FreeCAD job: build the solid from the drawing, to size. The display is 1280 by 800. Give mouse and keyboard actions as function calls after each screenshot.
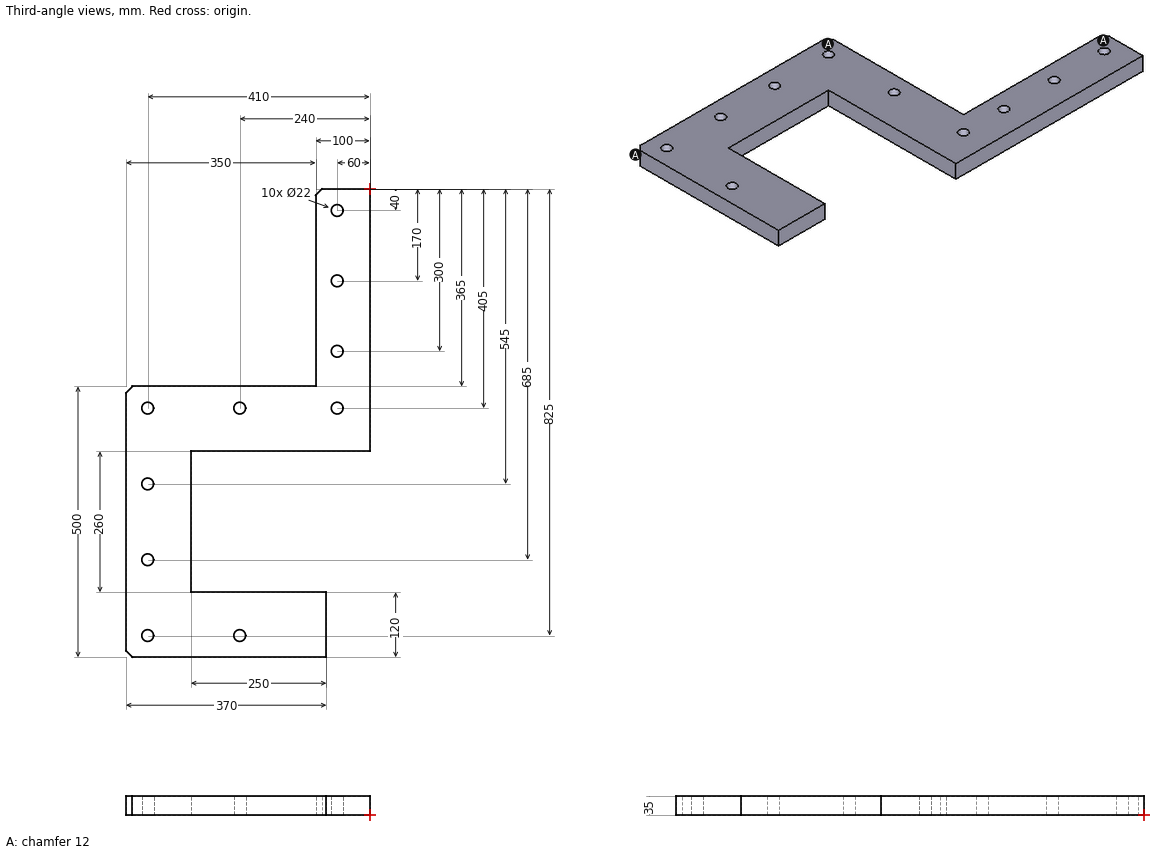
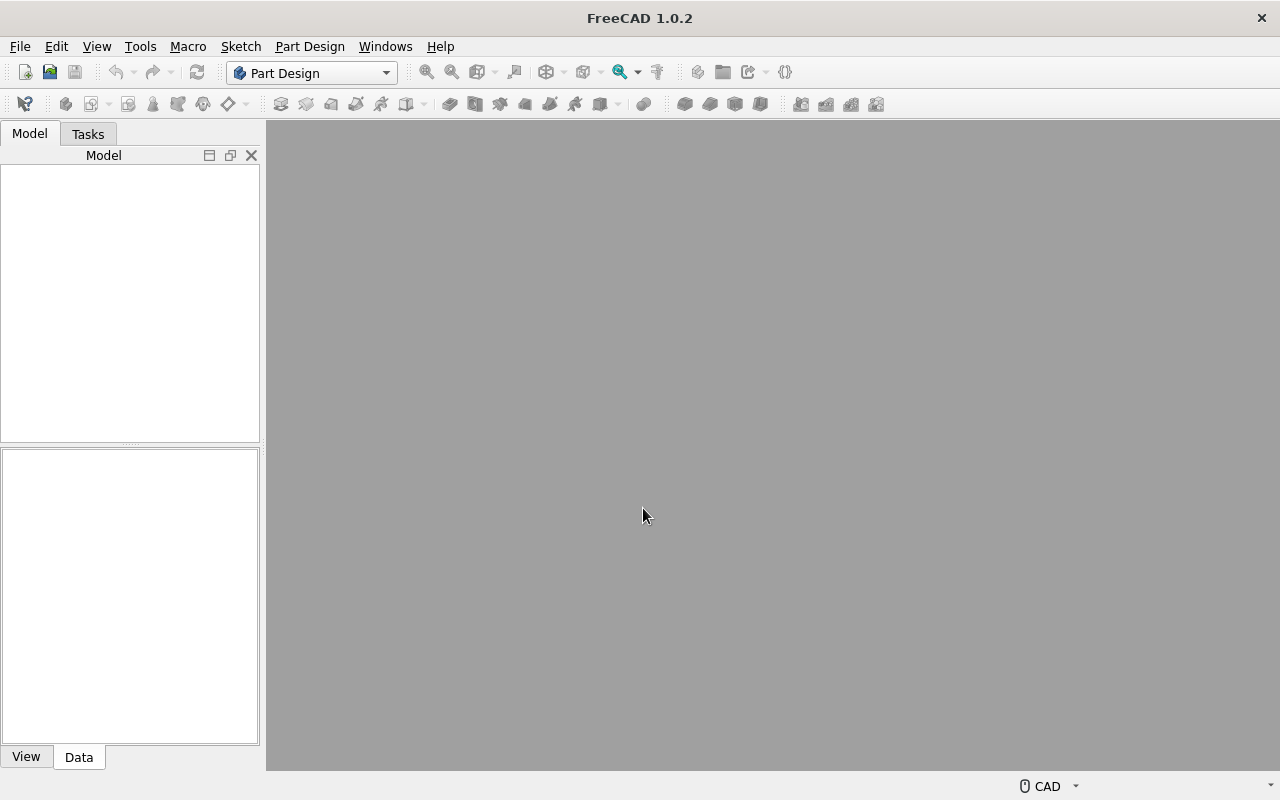
click(25, 72)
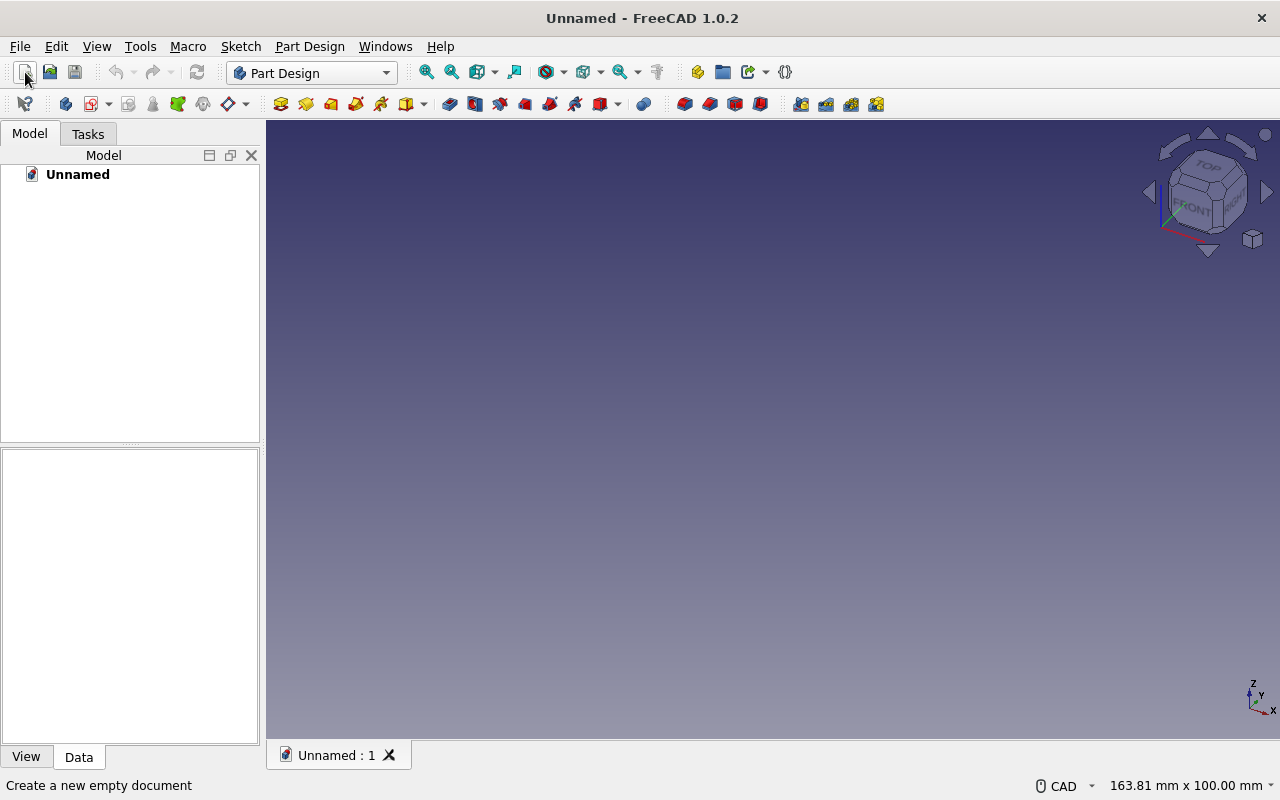
click(90, 104)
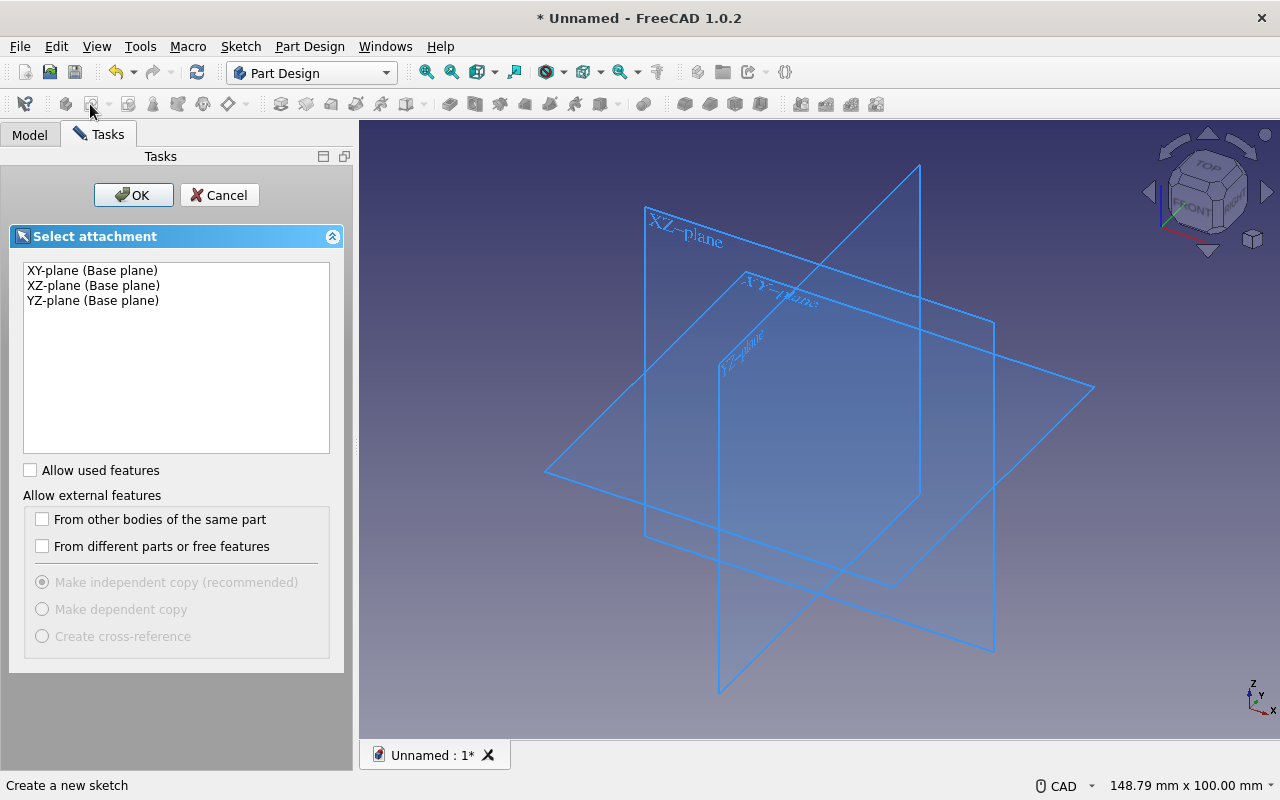
click(84, 270)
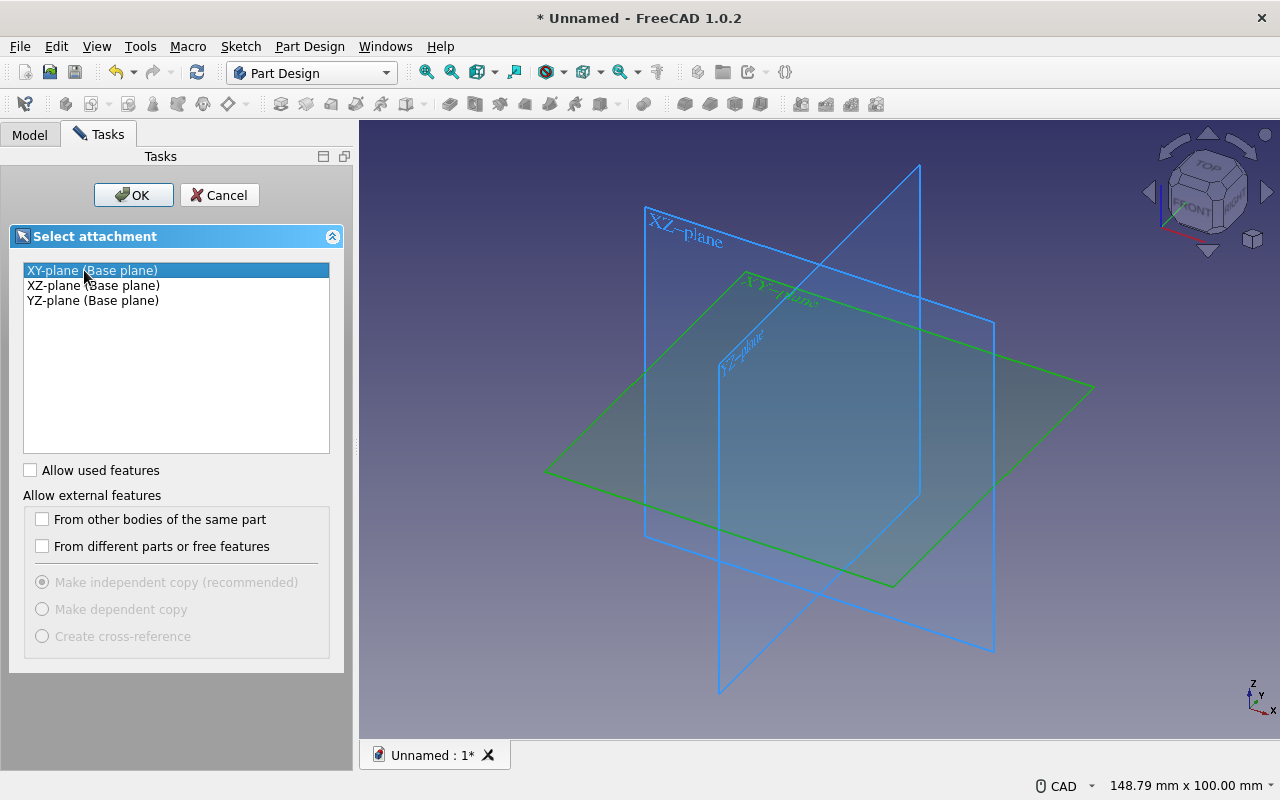
click(134, 195)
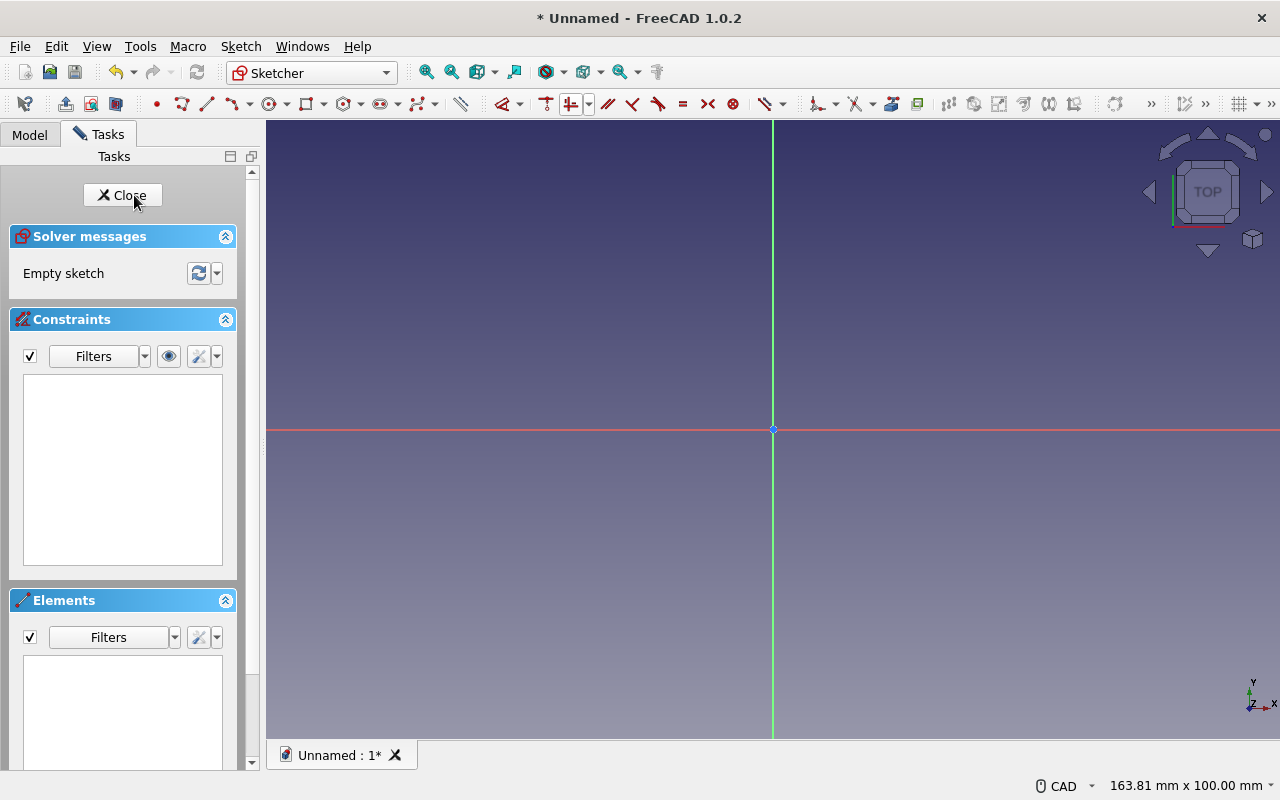
scroll(811, 215, down, 13)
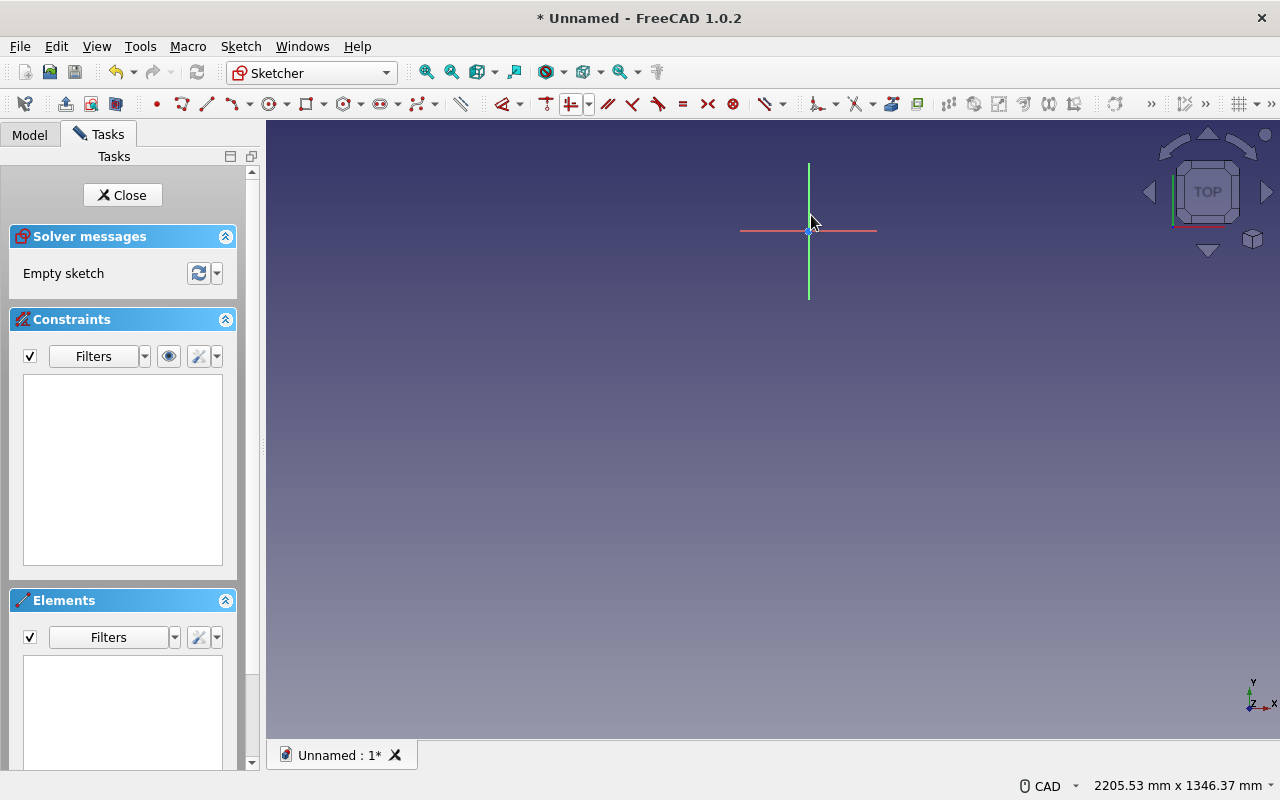
click(182, 104)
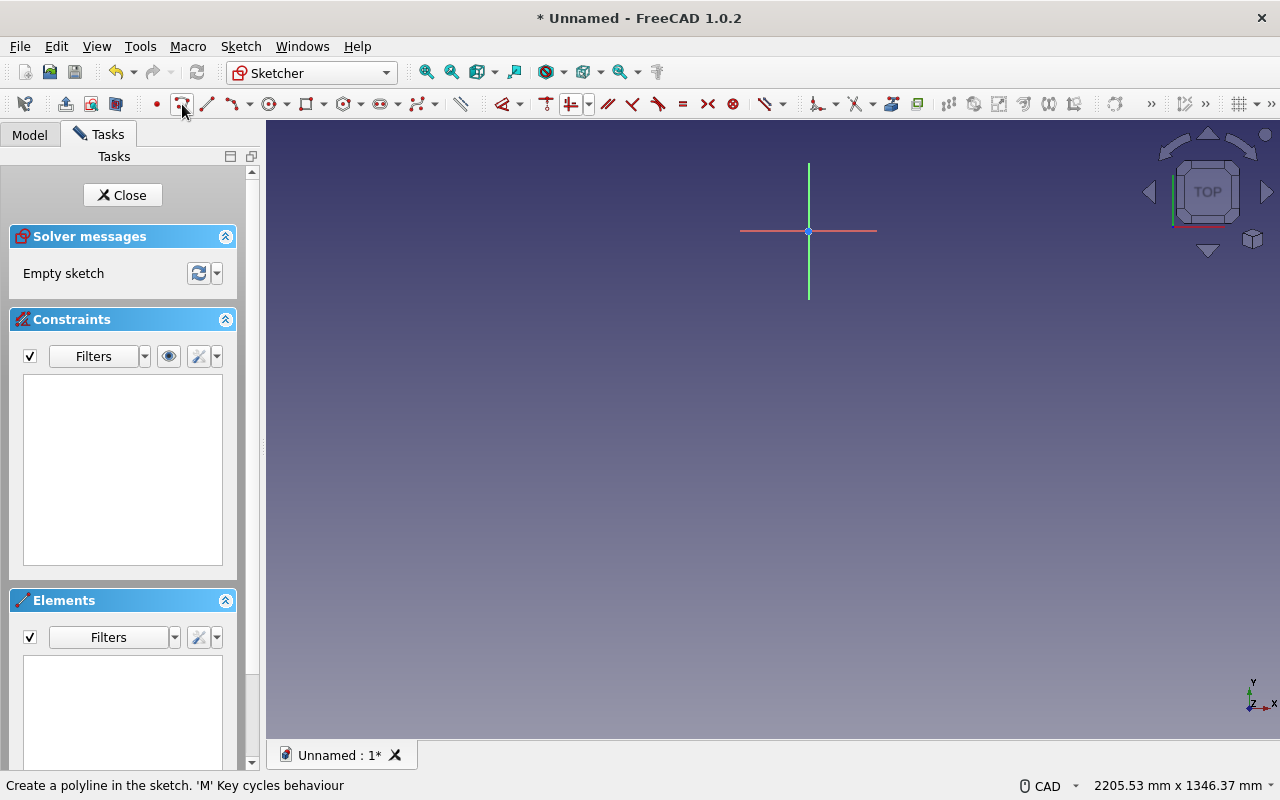
click(809, 231)
click(763, 240)
click(763, 399)
click(602, 399)
click(602, 629)
click(772, 629)
click(772, 574)
click(657, 574)
click(657, 454)
click(800, 454)
click(809, 231)
key(Escape)
key(Escape)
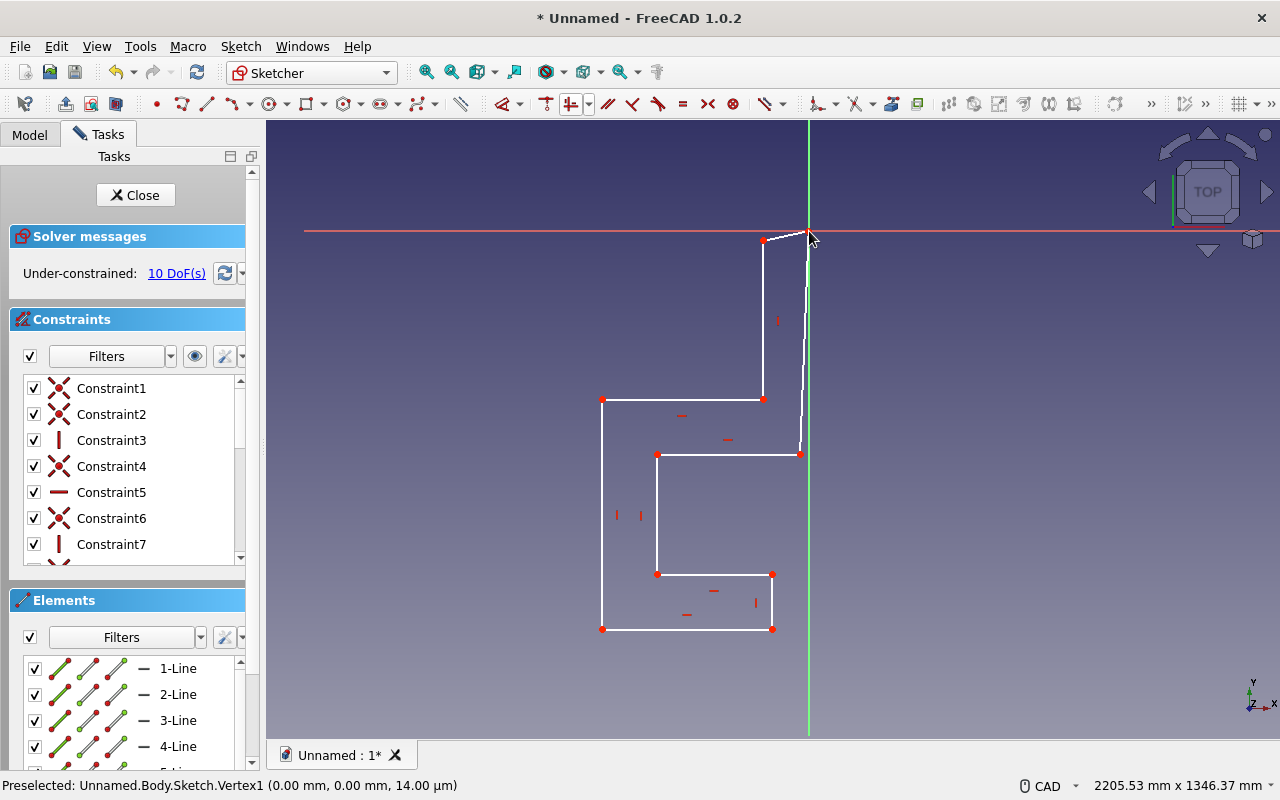
click(795, 234)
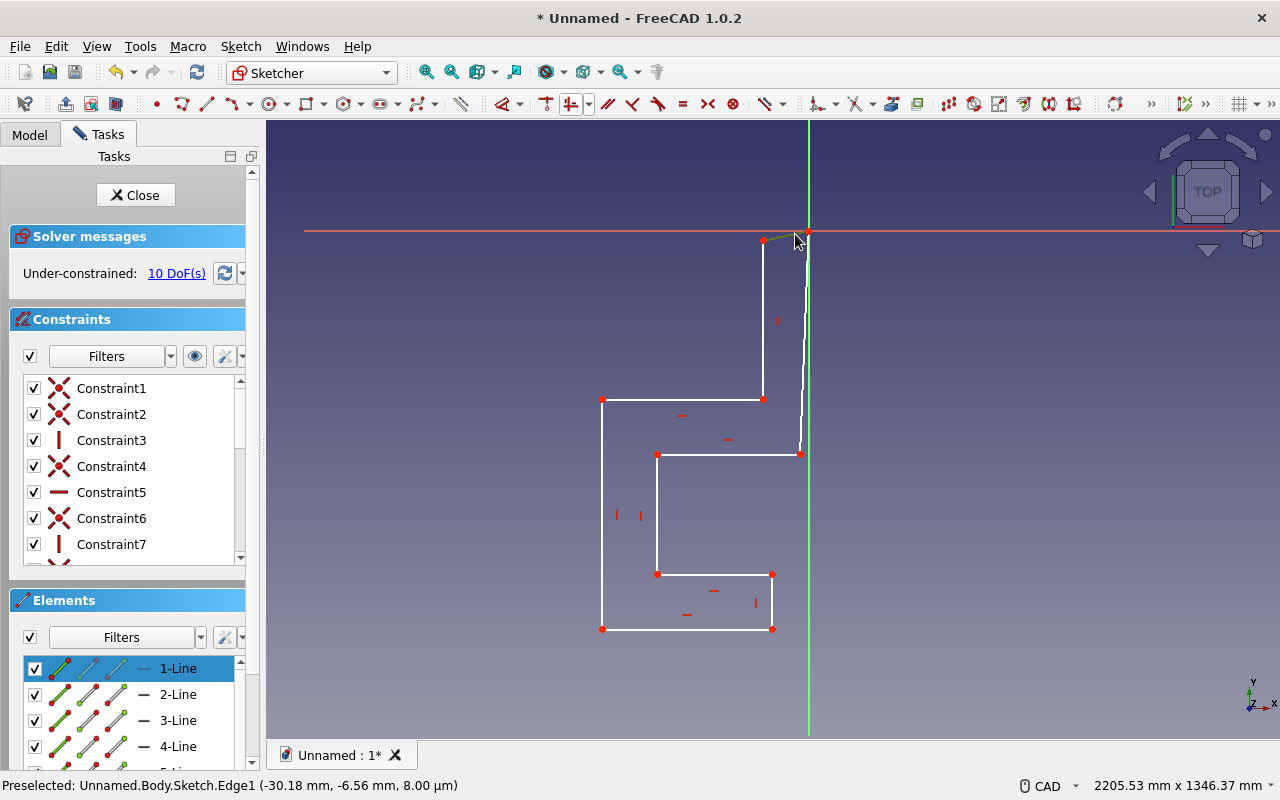
click(588, 104)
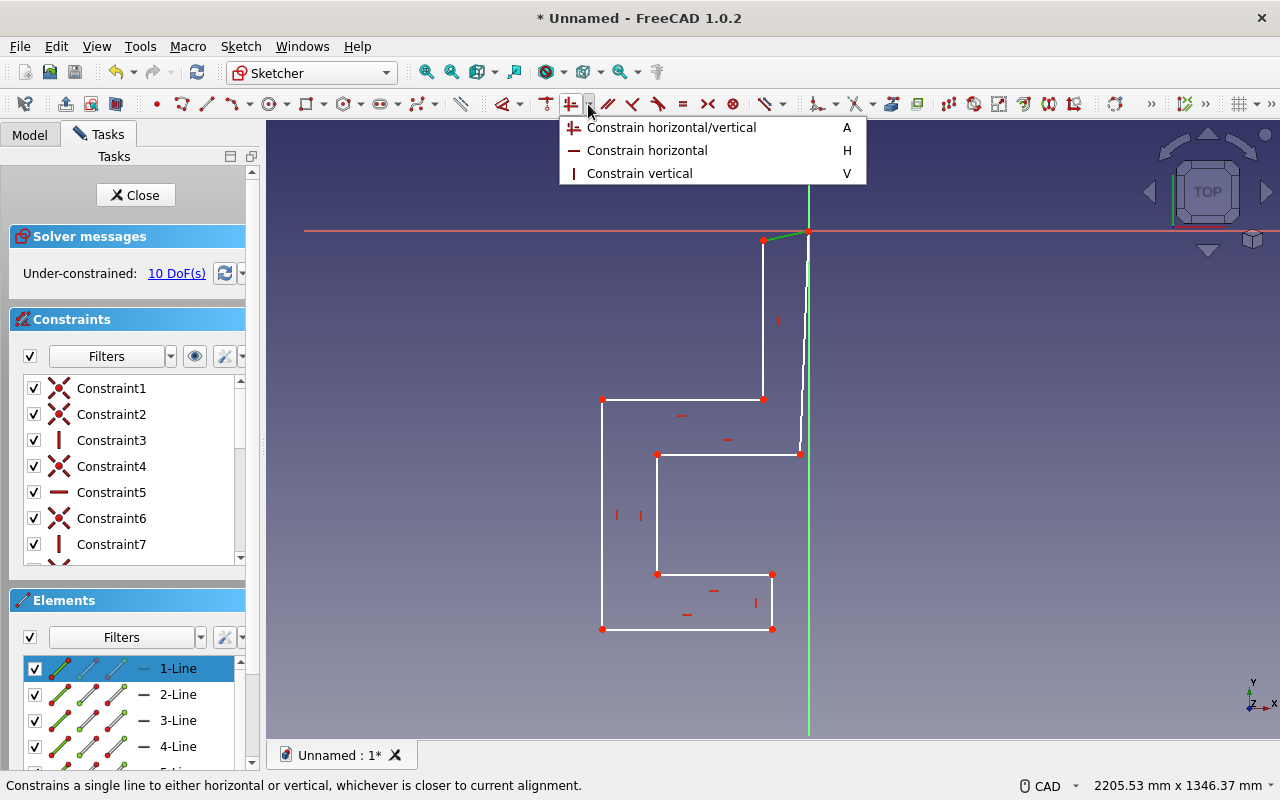
click(713, 150)